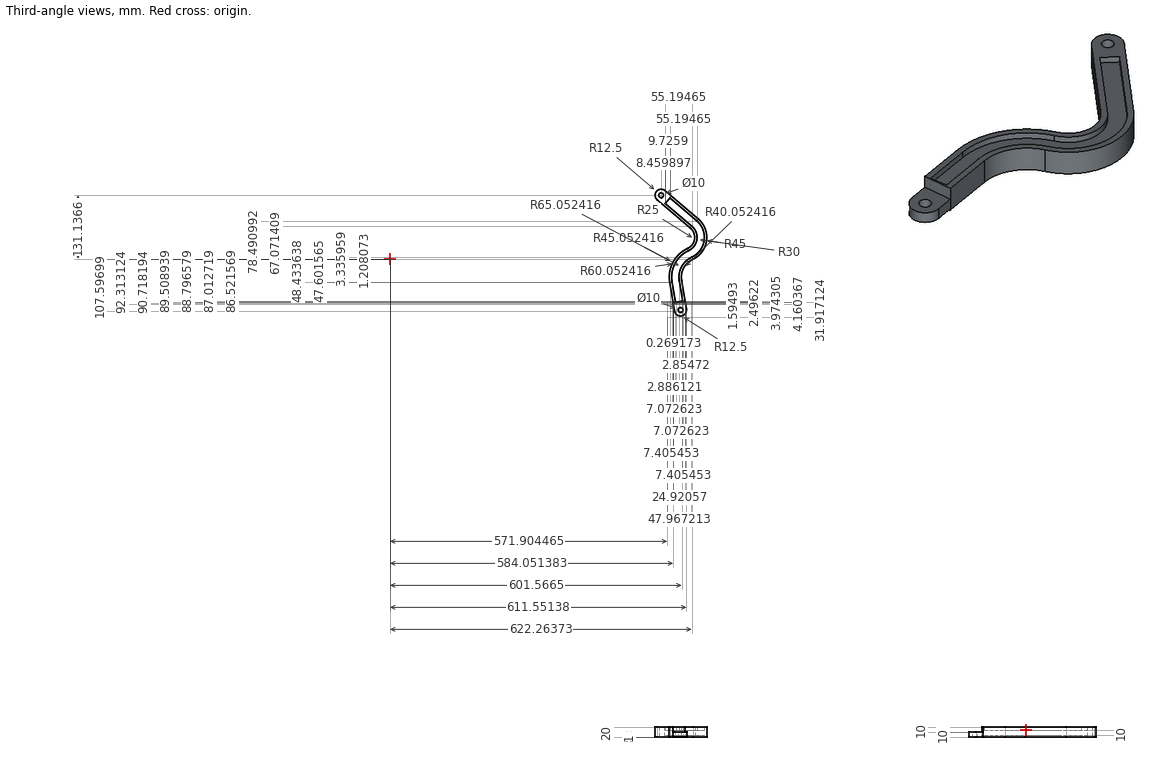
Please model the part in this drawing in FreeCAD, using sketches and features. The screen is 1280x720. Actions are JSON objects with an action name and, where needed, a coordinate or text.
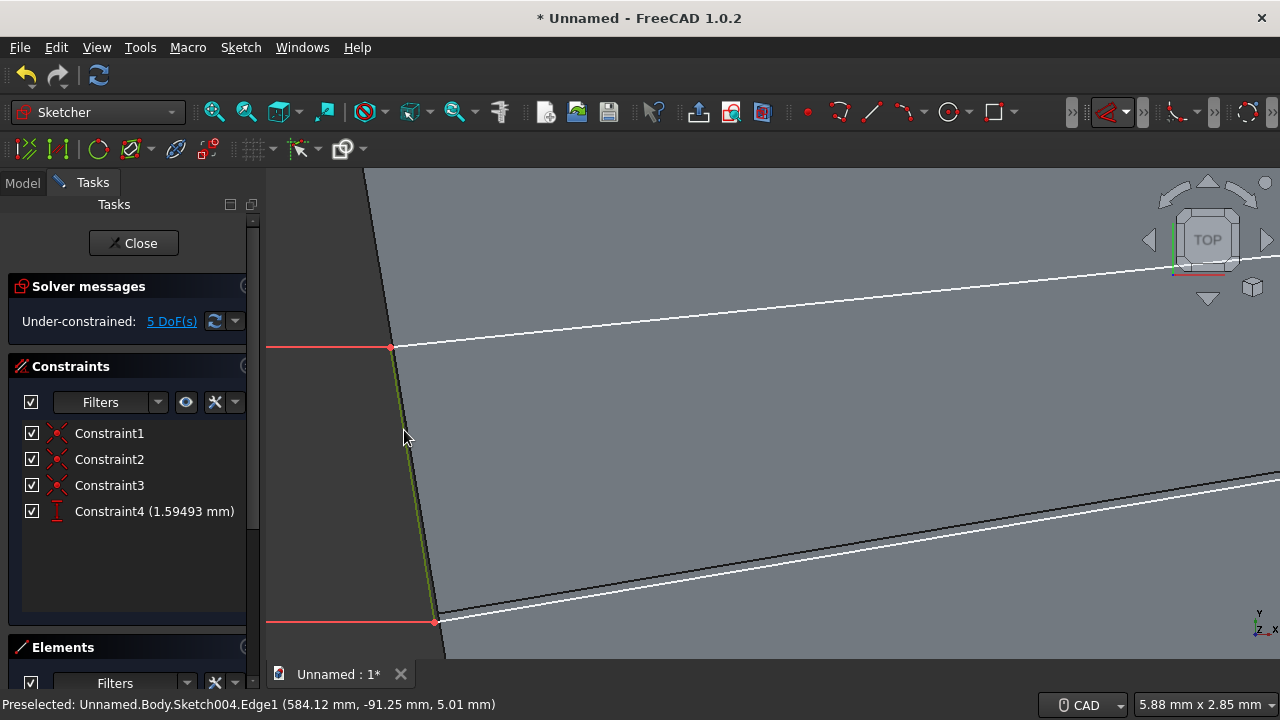
{"action": "key", "text": "l"}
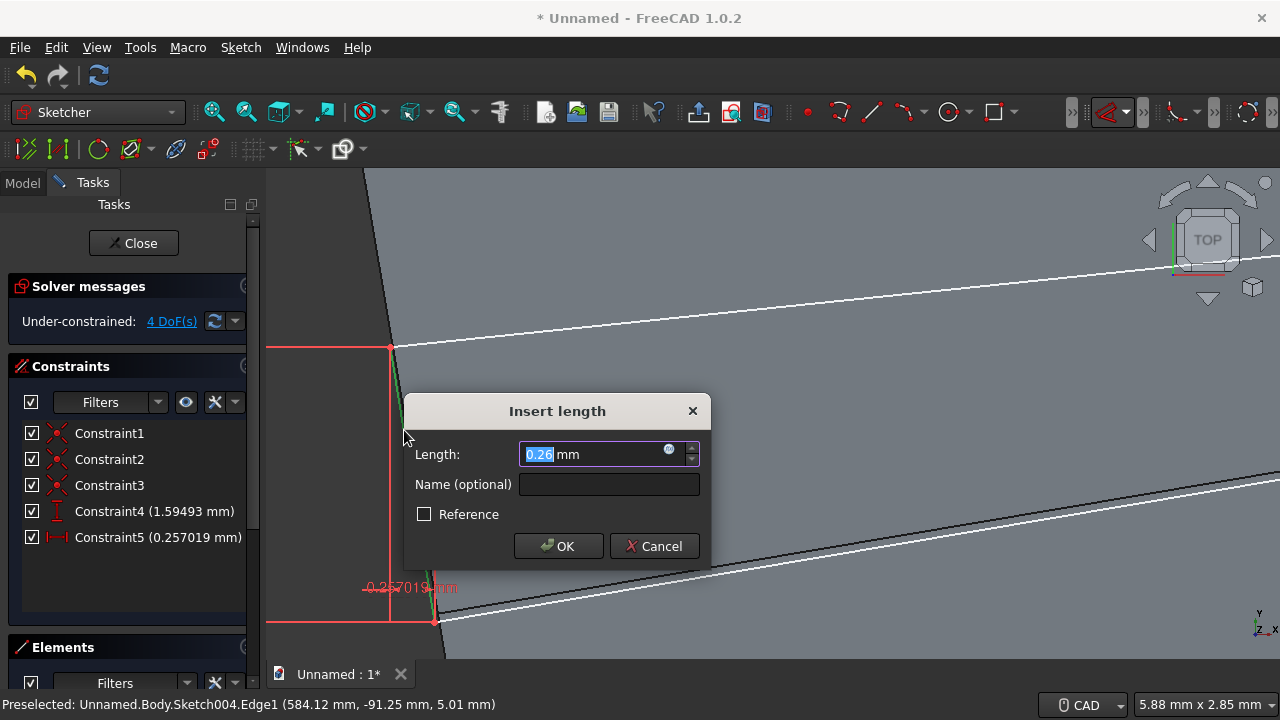
{"action": "type", "text": "0.269173"}
{"action": "key", "text": "Return"}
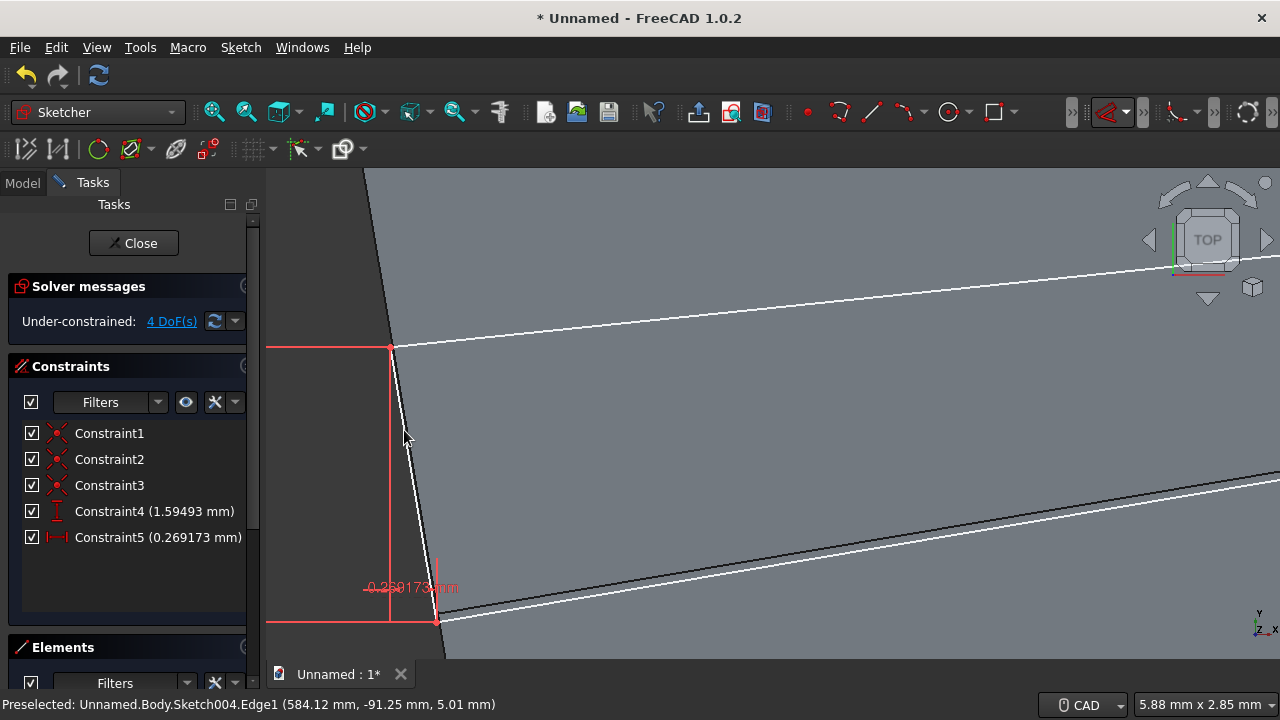
{"action": "scroll", "coordinate": [417, 438], "scroll_direction": "down", "scroll_amount": 10}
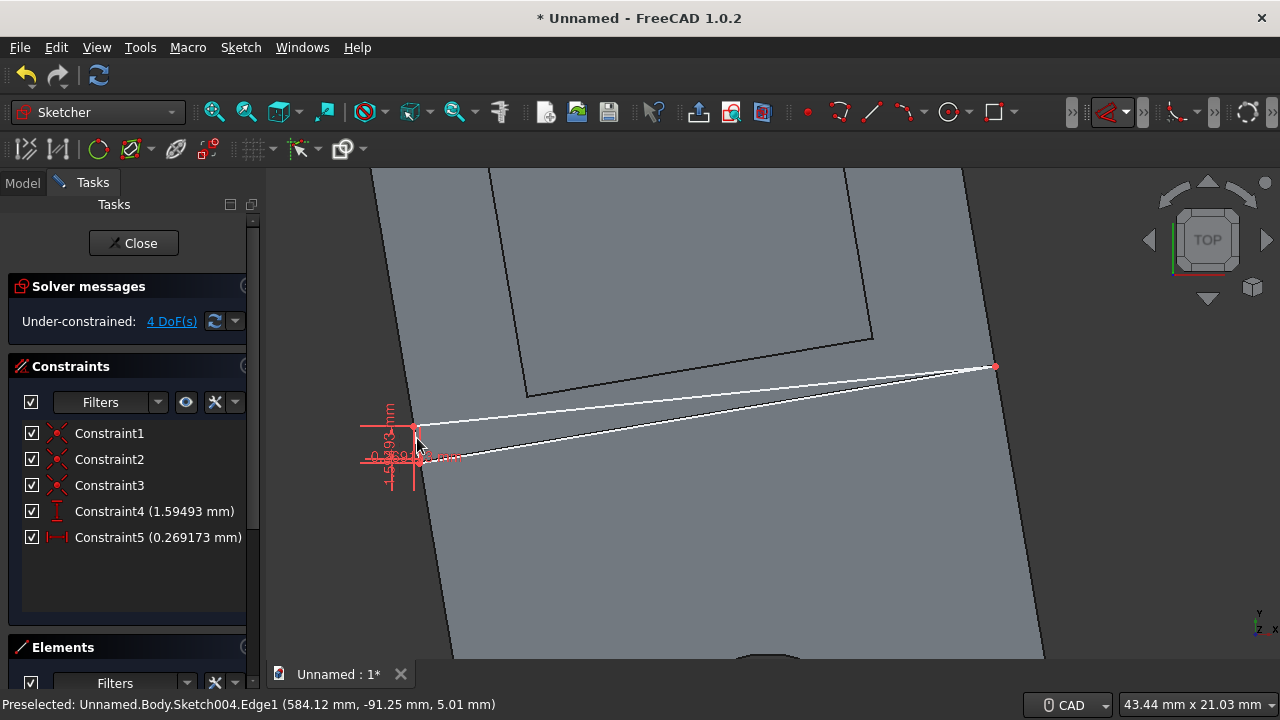
{"action": "left_click", "coordinate": [593, 434]}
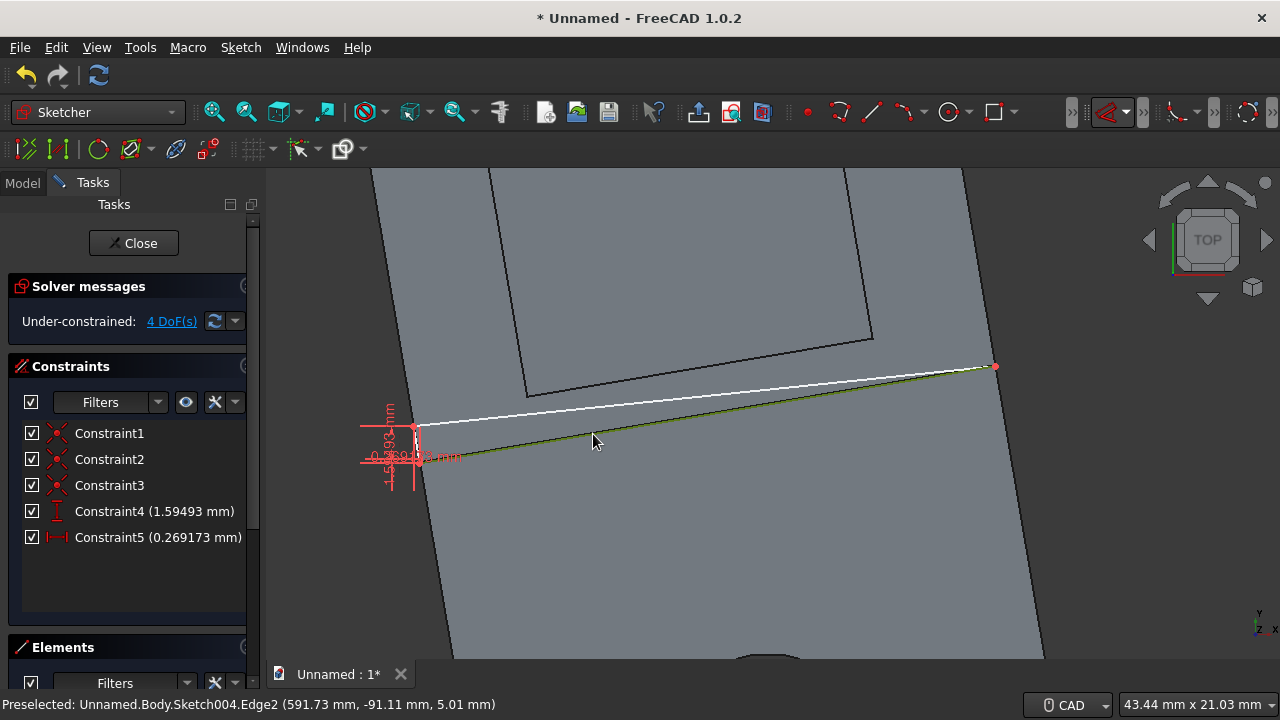
{"action": "key", "text": "i"}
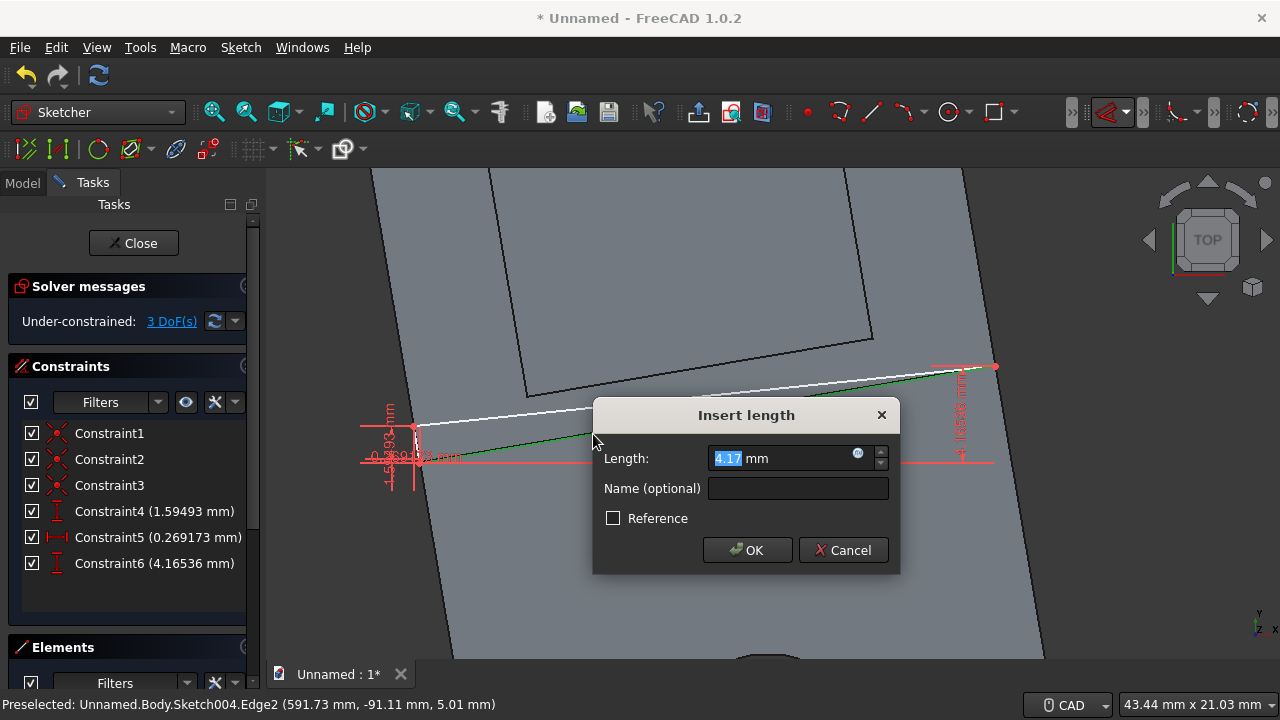
{"action": "type", "text": "4.160367"}
{"action": "key", "text": "Return"}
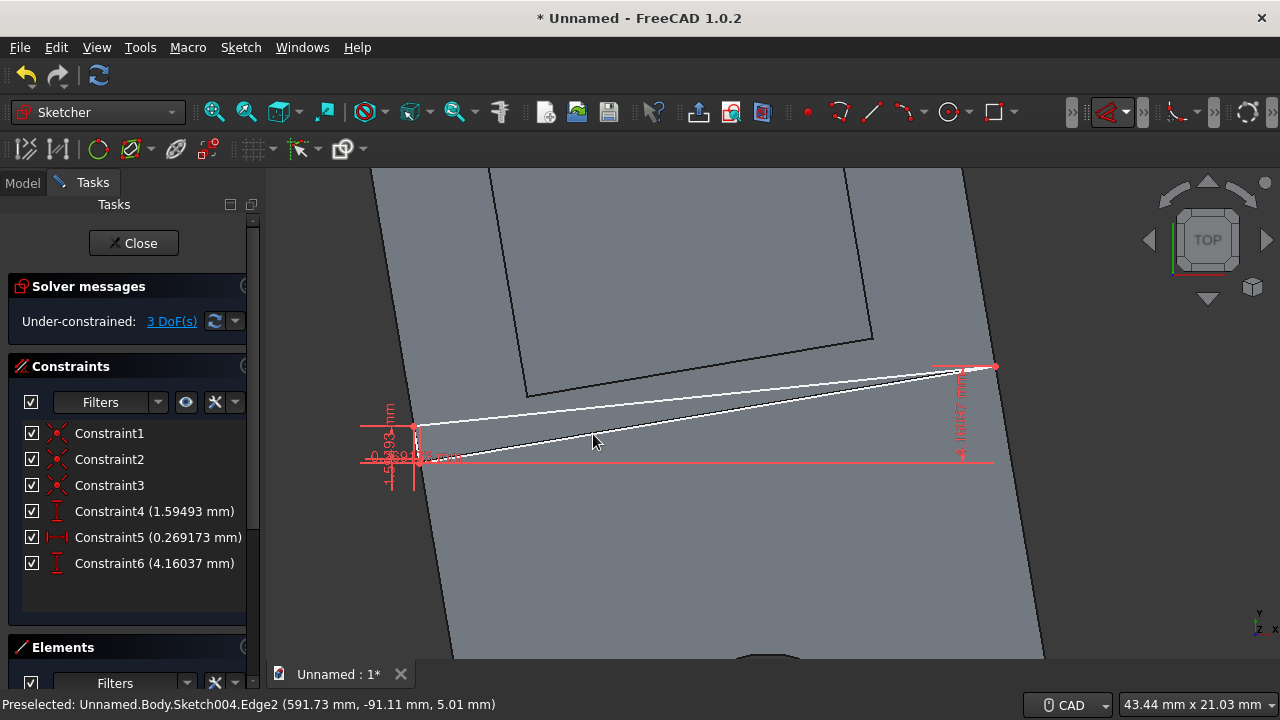
{"action": "left_click", "coordinate": [821, 384]}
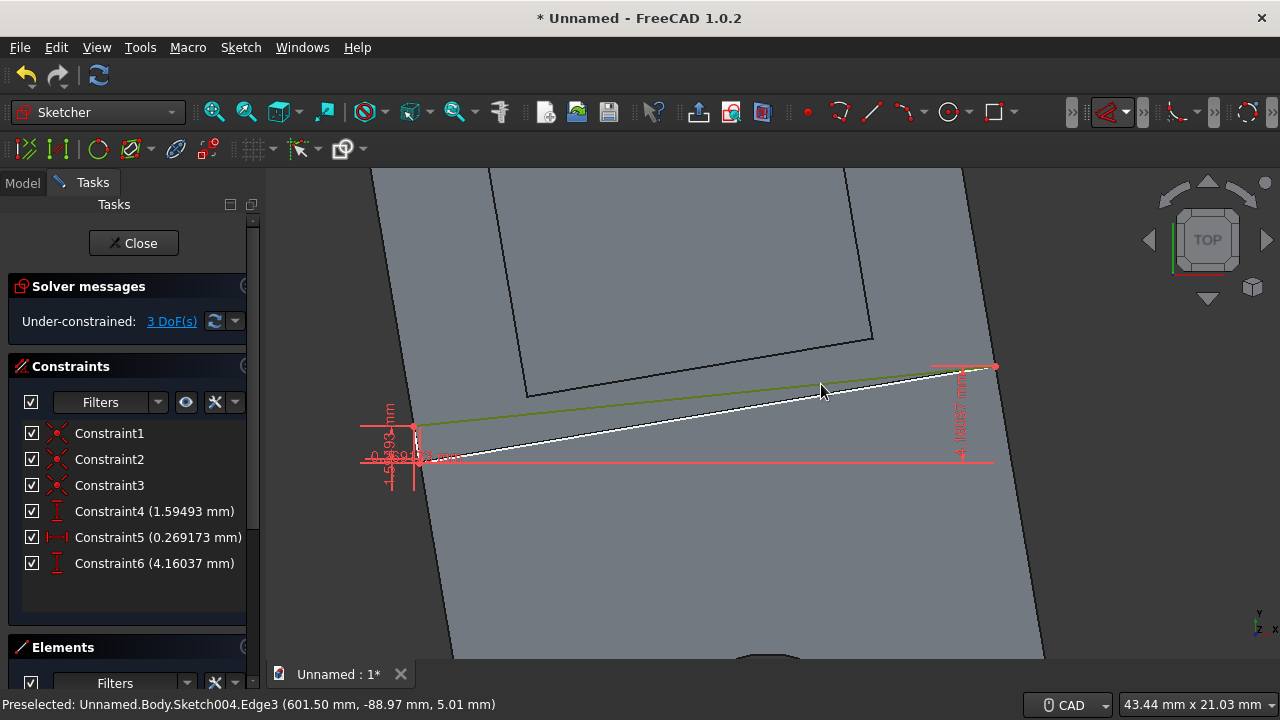
{"action": "key", "text": "l"}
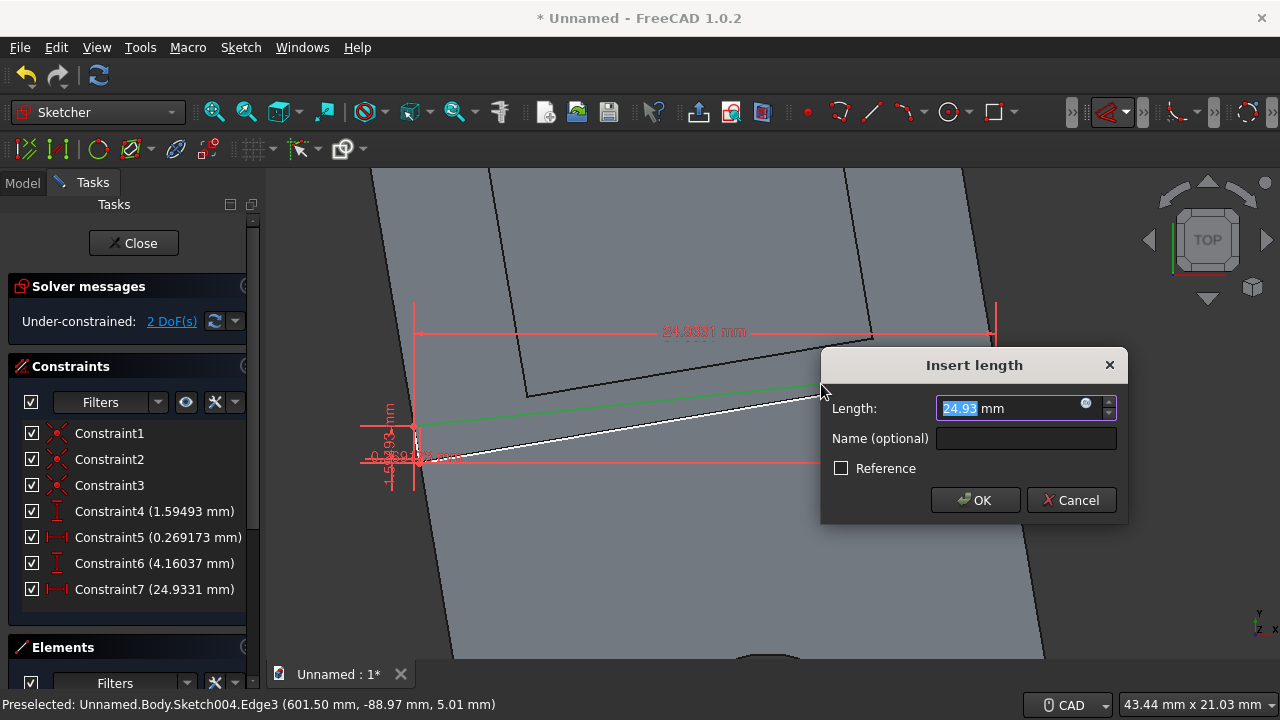
{"action": "type", "text": "24.92057"}
{"action": "key", "text": "Return"}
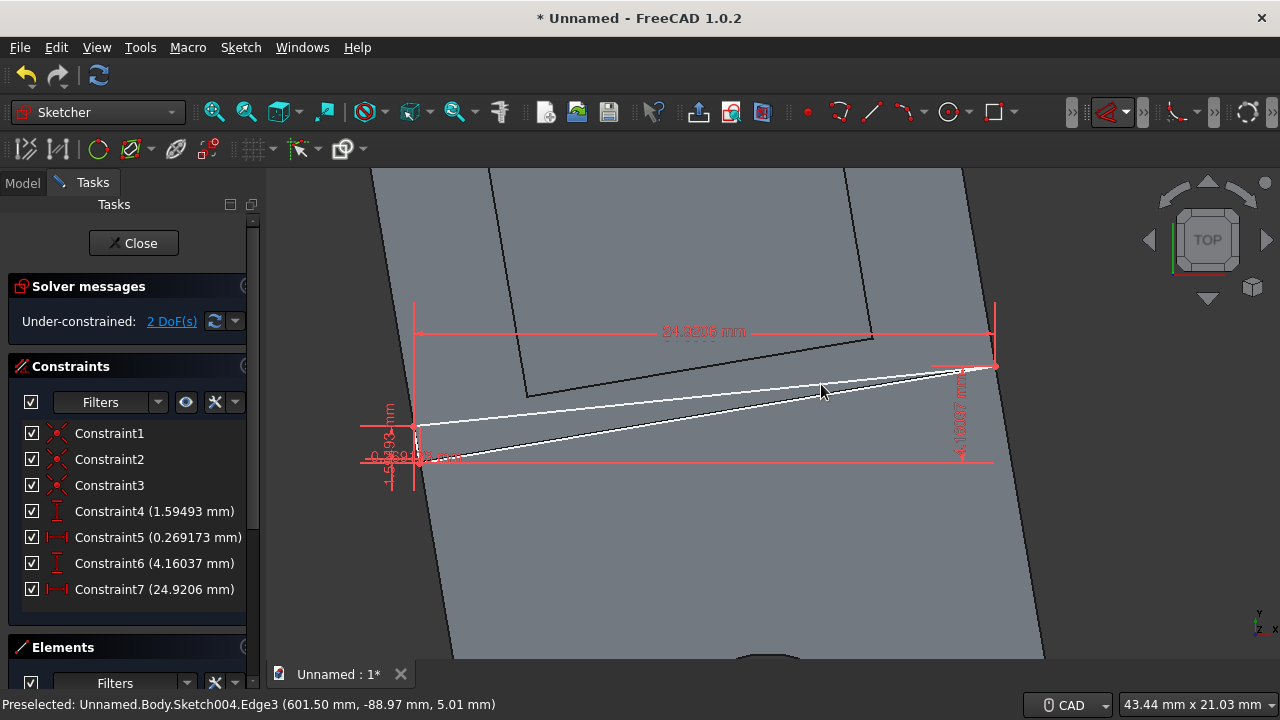
{"action": "left_click", "coordinate": [414, 426]}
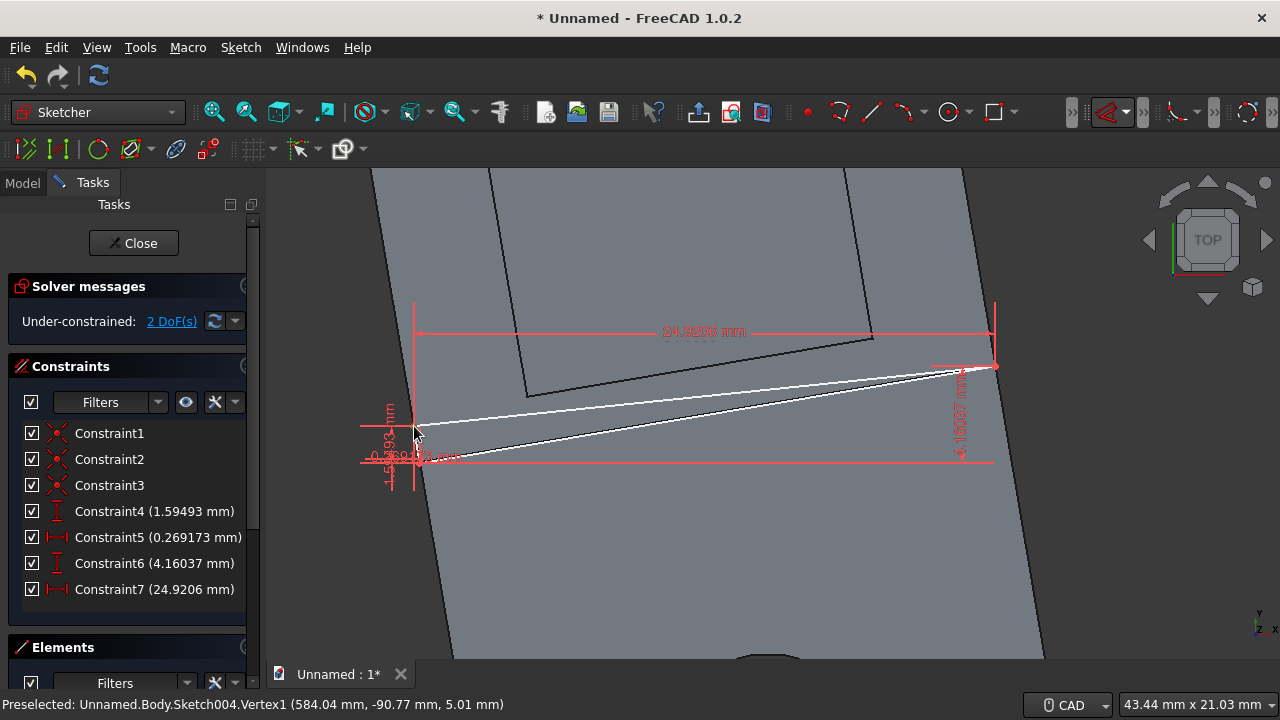
{"action": "key", "text": "i"}